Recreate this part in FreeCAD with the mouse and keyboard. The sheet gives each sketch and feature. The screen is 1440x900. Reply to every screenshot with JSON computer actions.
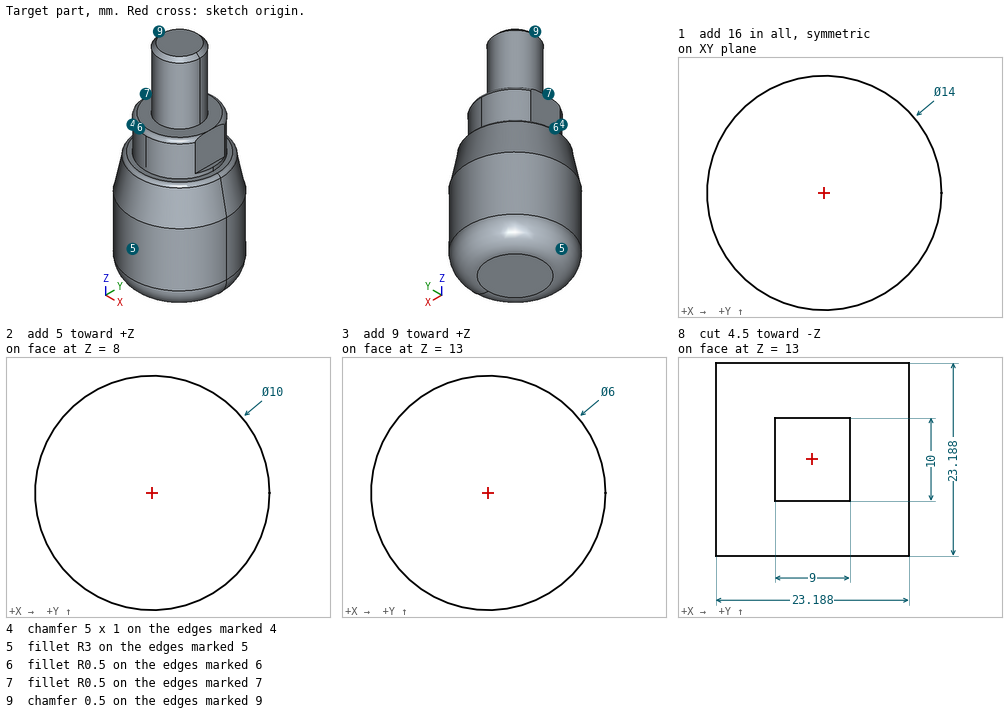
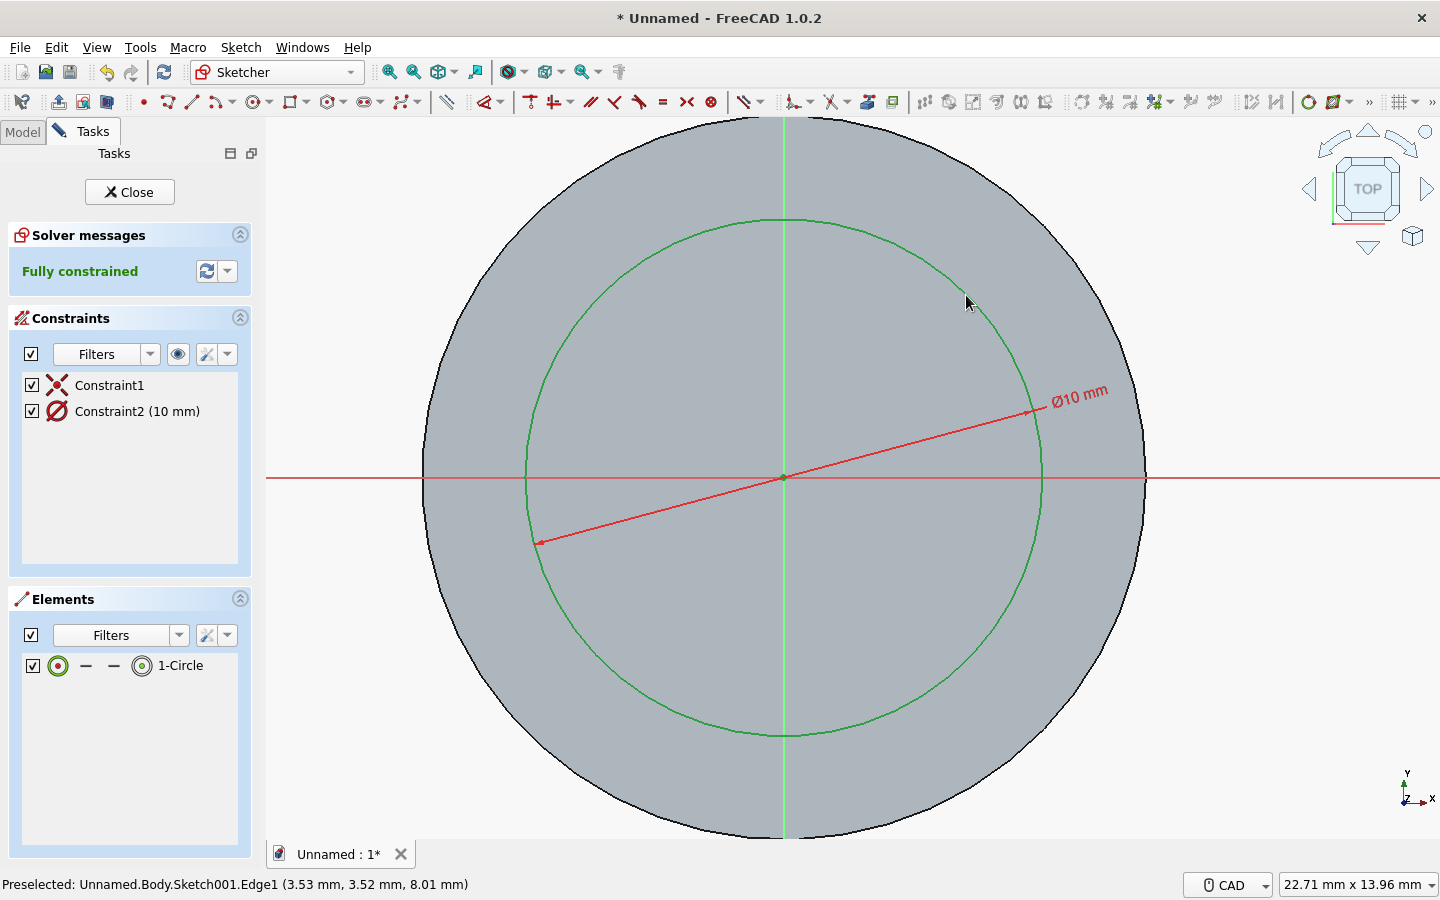
{"action": "left_click", "coordinate": [130, 192]}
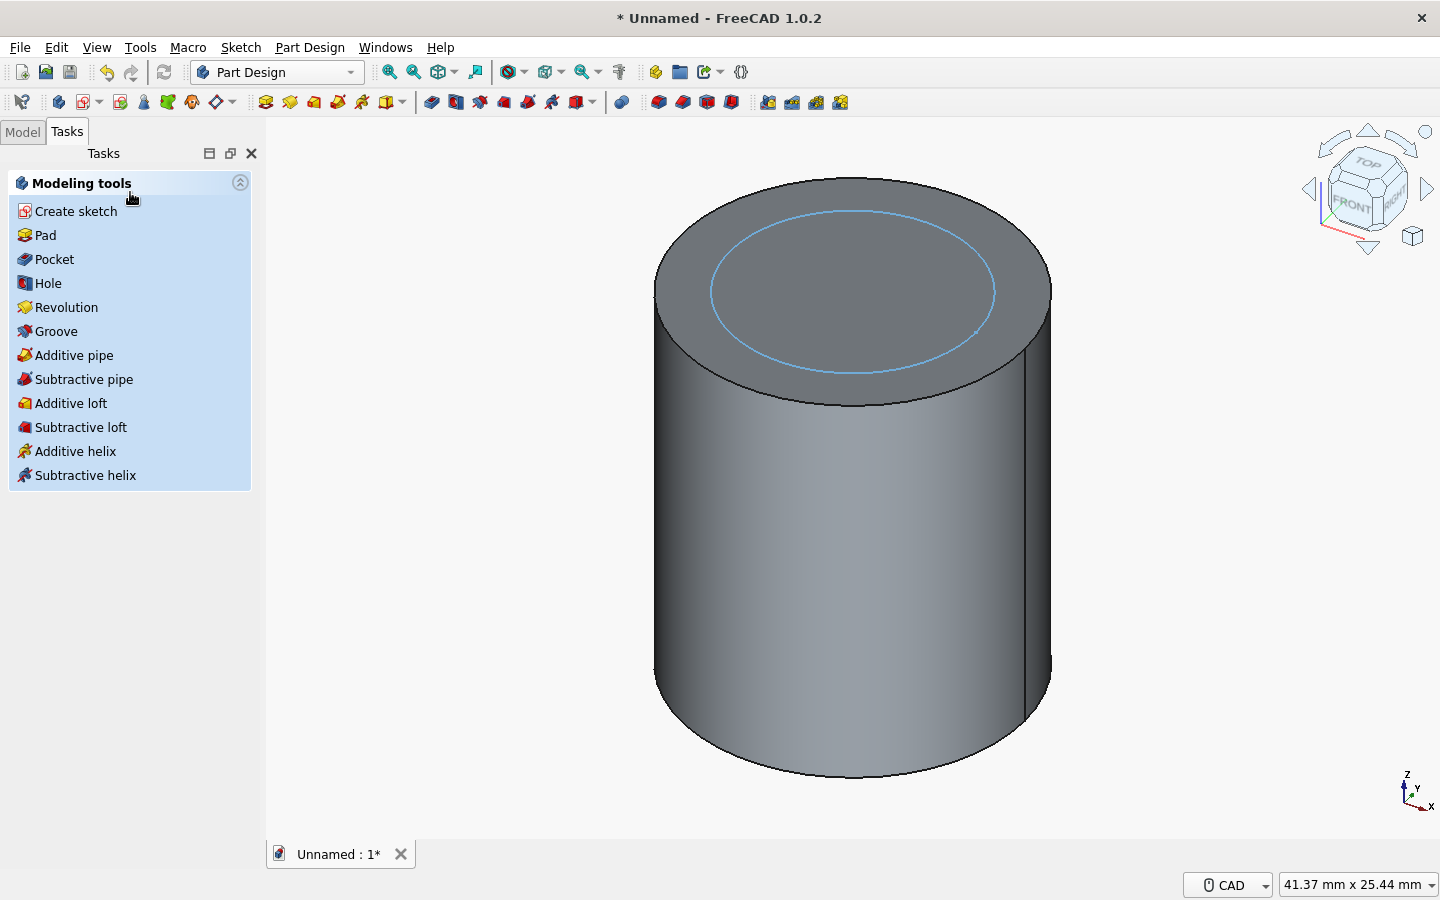
{"action": "left_click", "coordinate": [266, 102]}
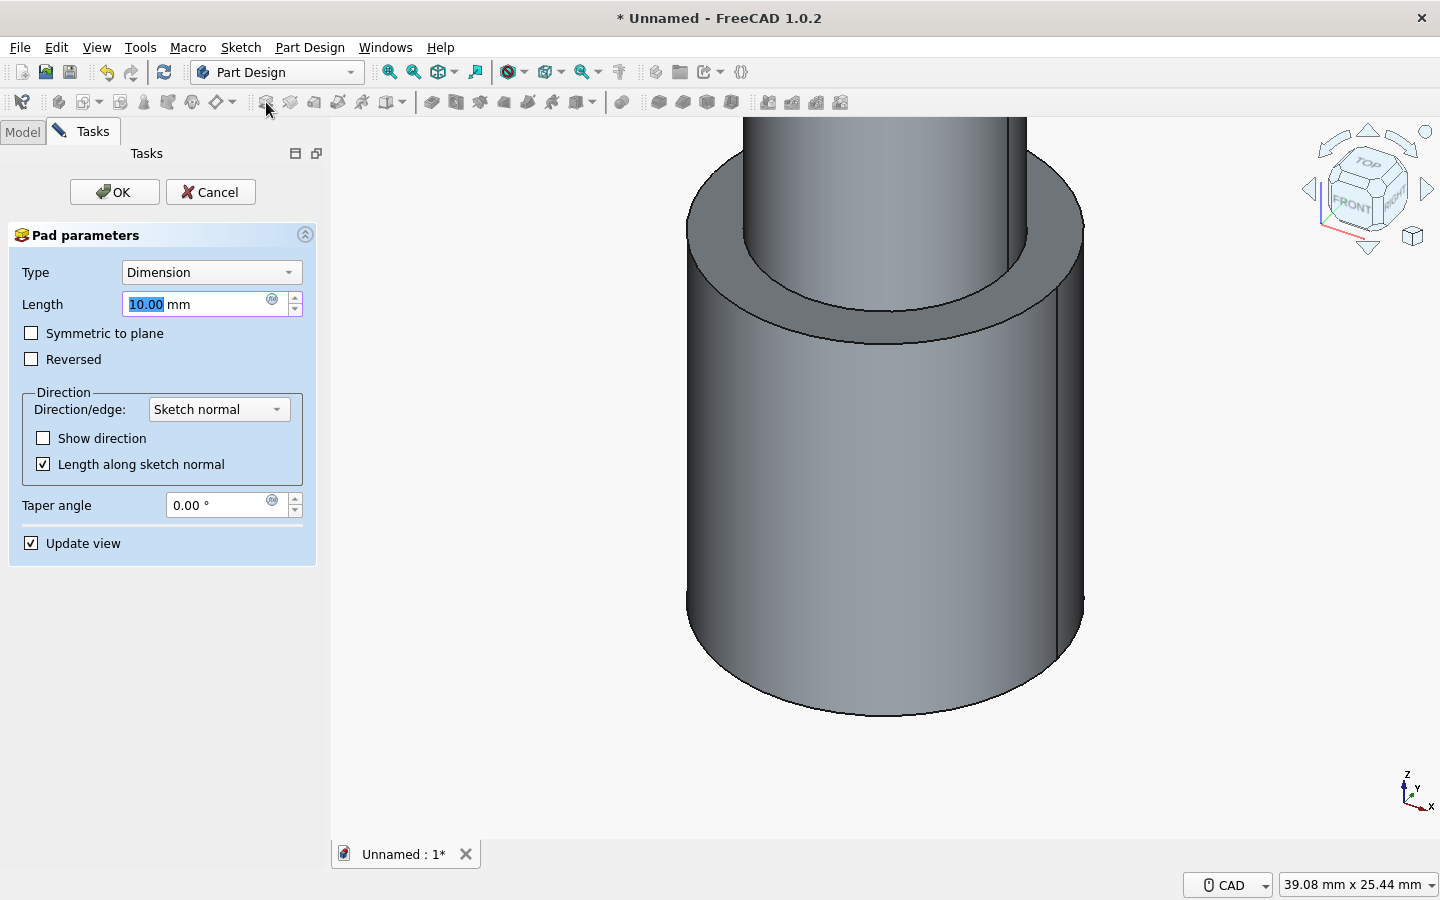
{"action": "type", "text": "5"}
{"action": "key", "text": "Tab"}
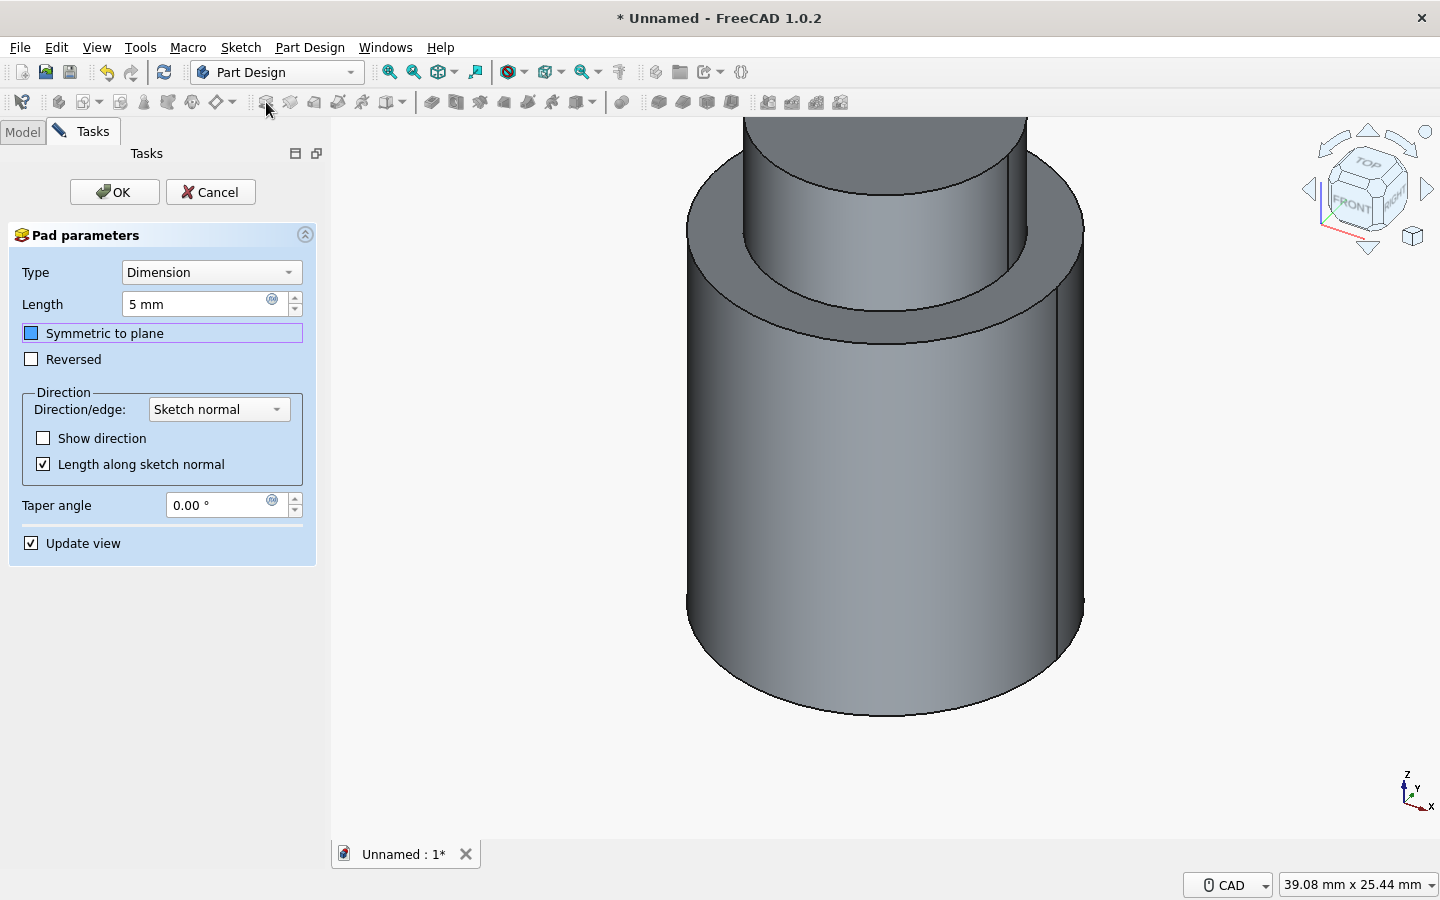
{"action": "left_click", "coordinate": [115, 192]}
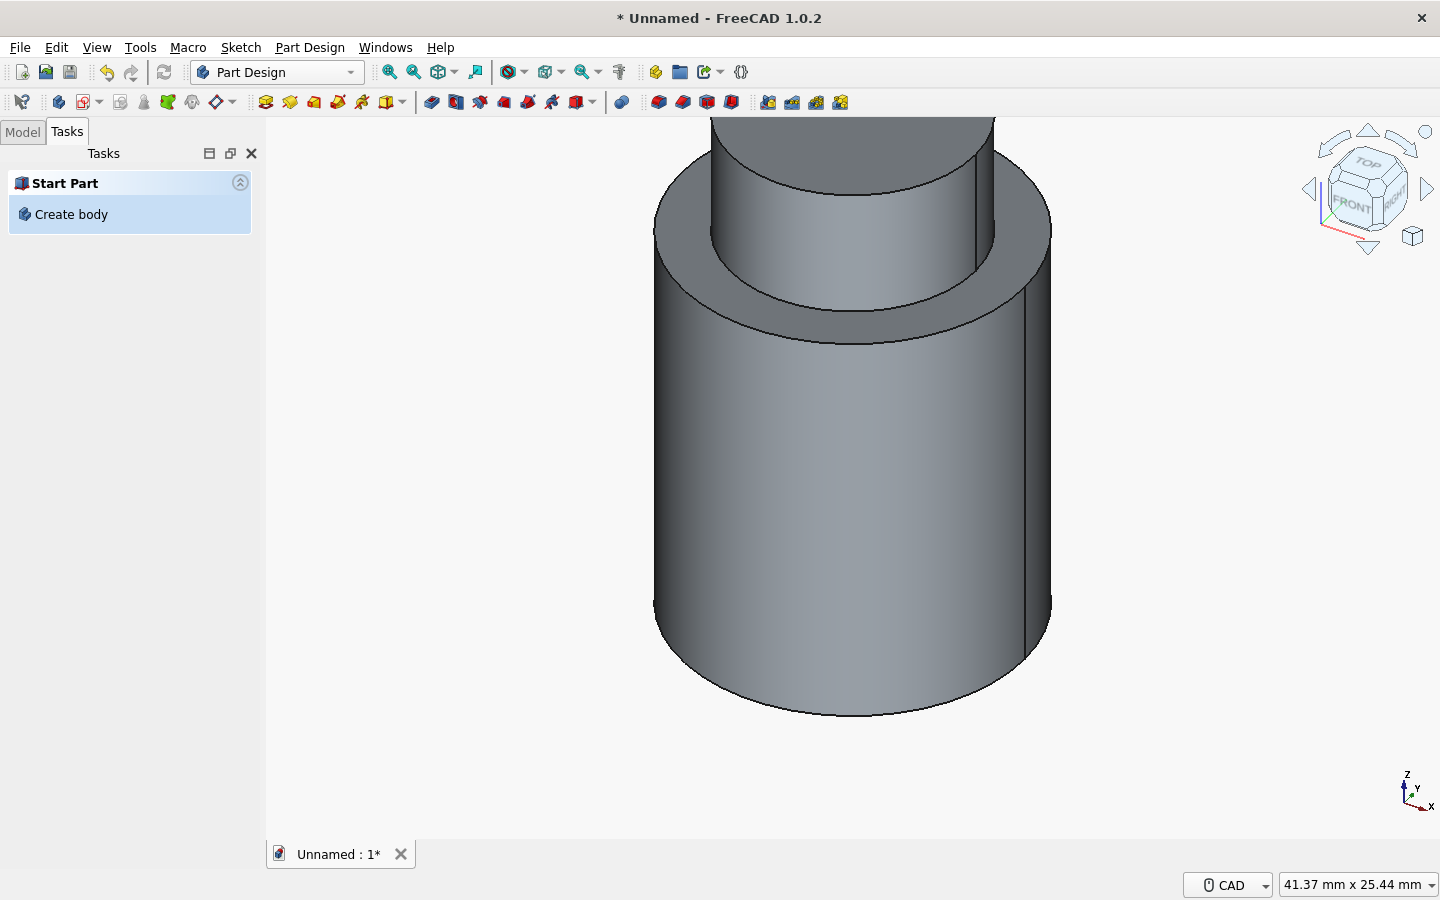
{"action": "key", "text": "v f"}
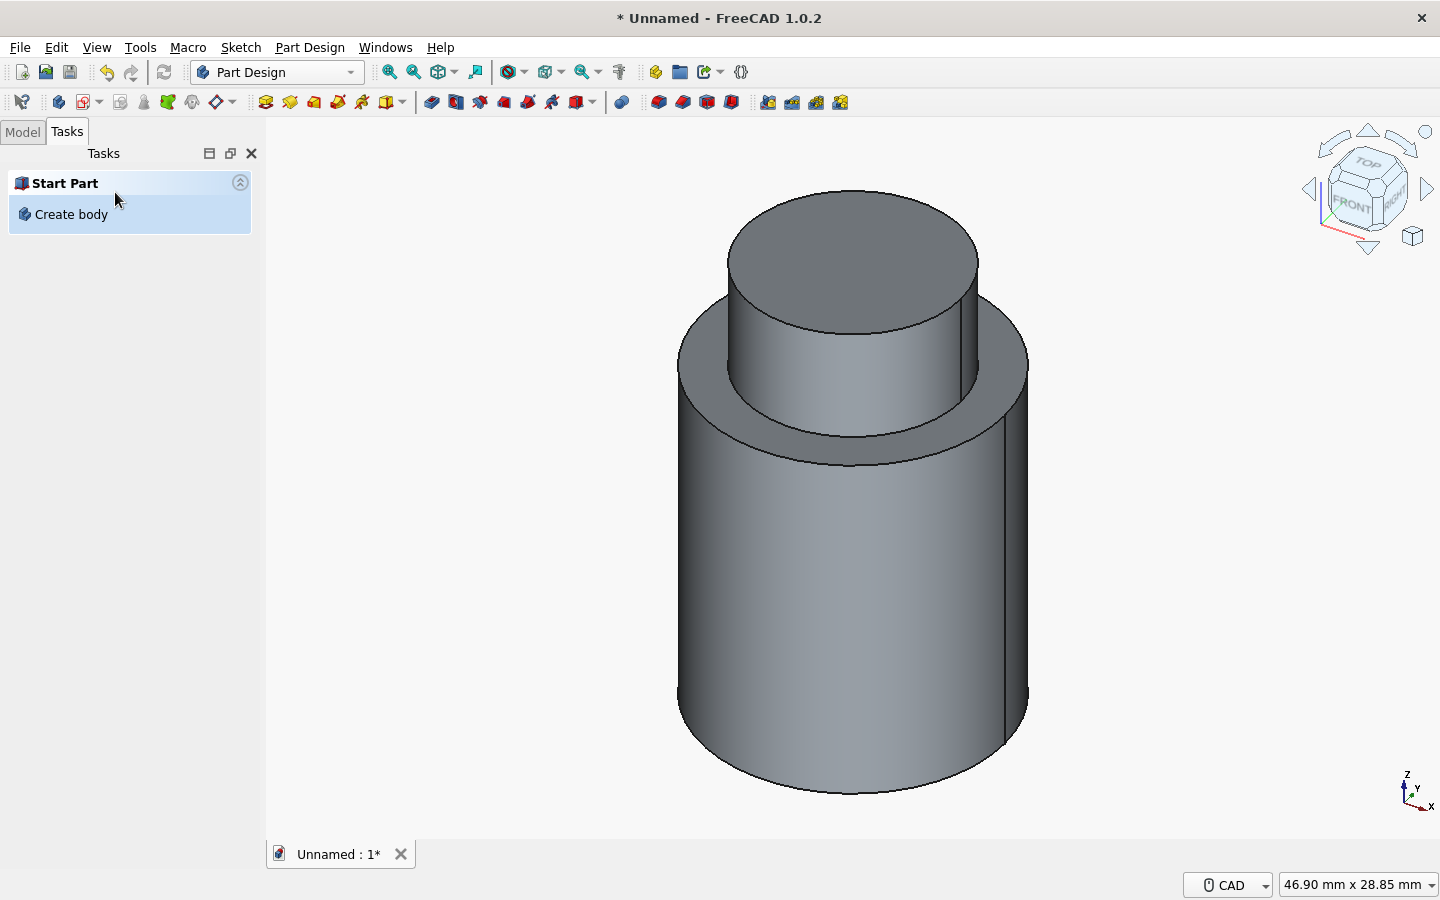
{"action": "left_click", "coordinate": [853, 262]}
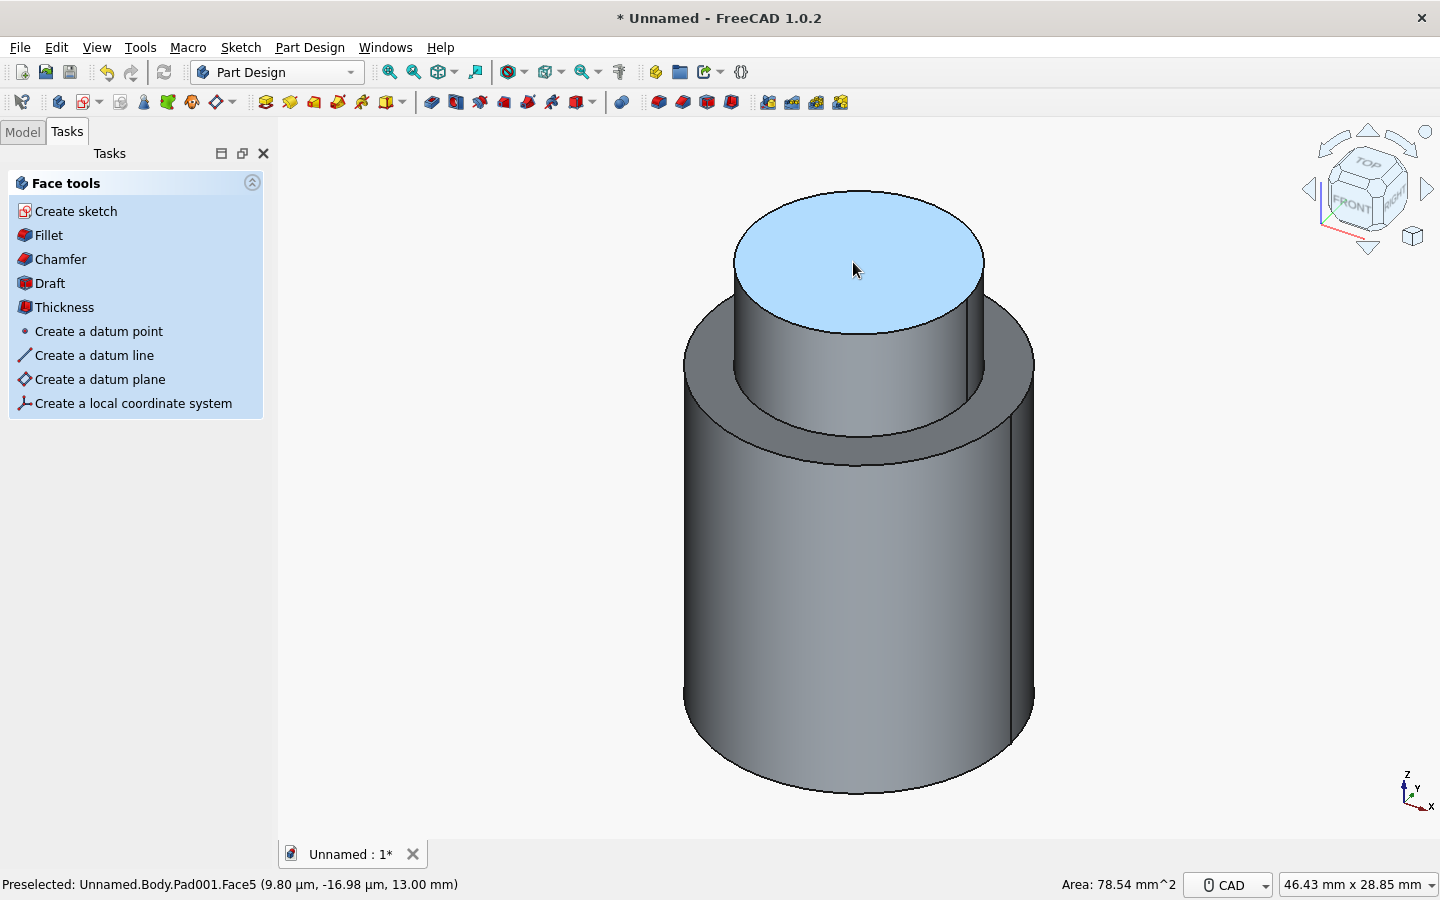
{"action": "left_click", "coordinate": [84, 102]}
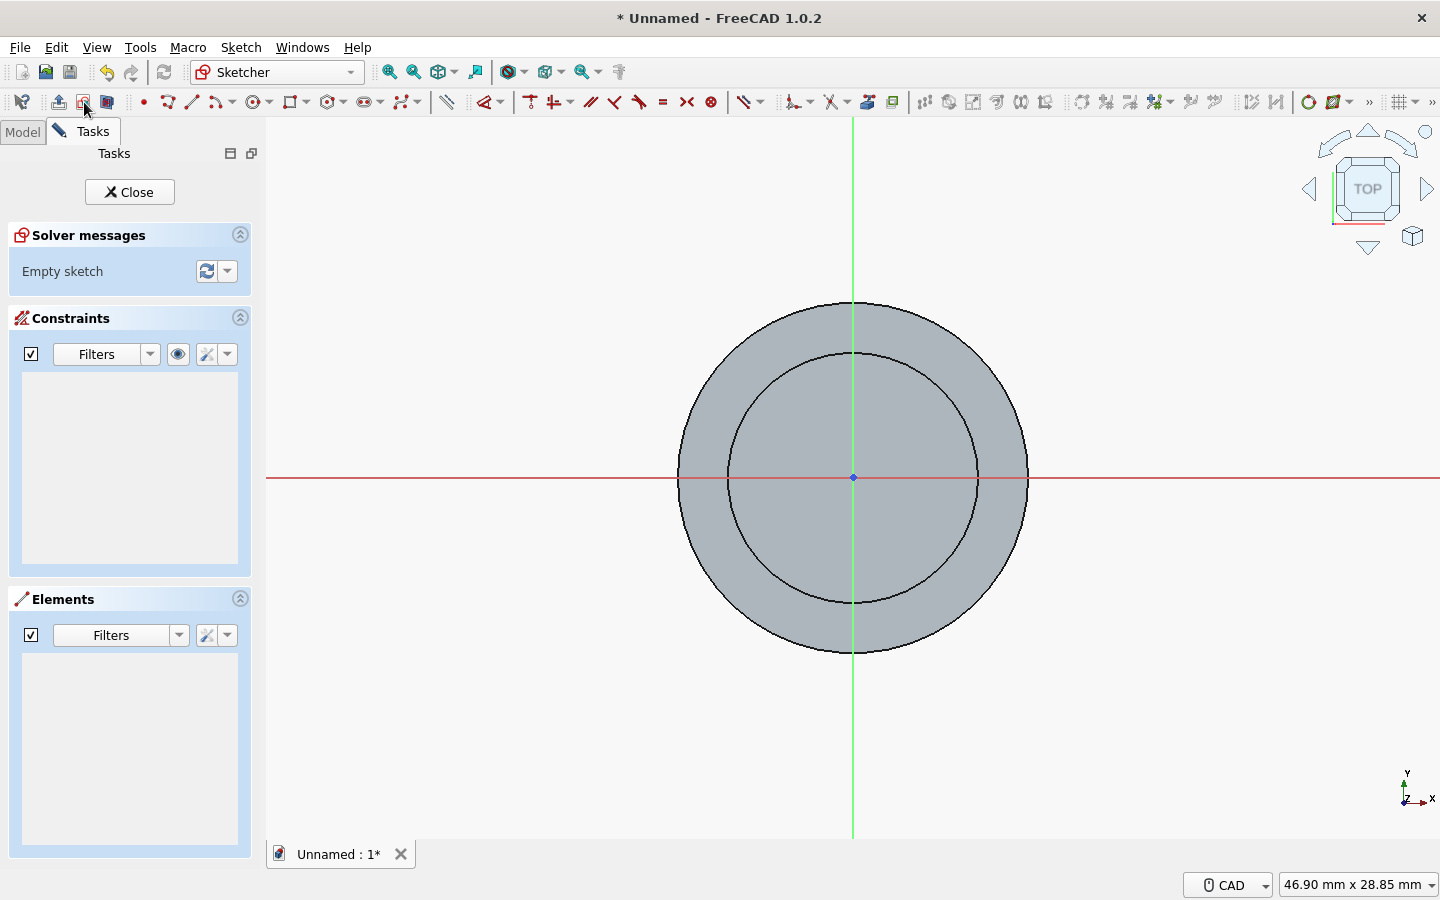
{"action": "scroll", "coordinate": [883, 478], "scroll_direction": "up", "scroll_amount": 6}